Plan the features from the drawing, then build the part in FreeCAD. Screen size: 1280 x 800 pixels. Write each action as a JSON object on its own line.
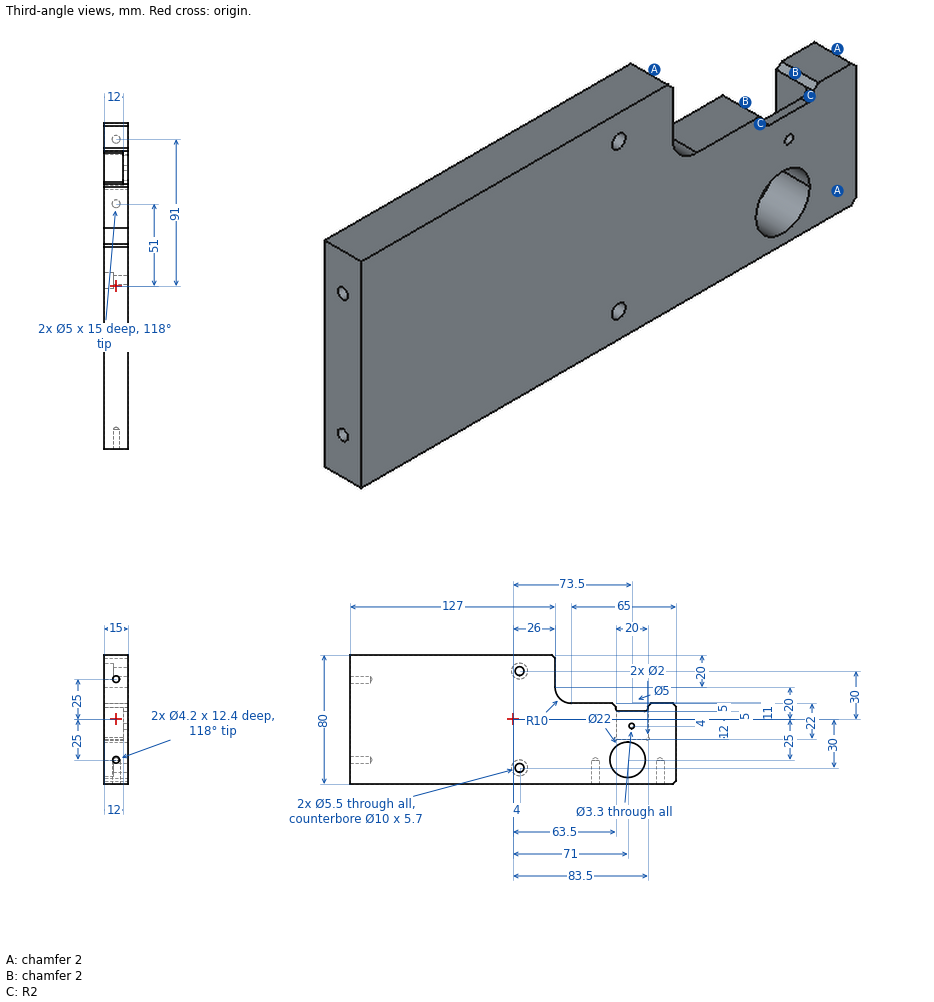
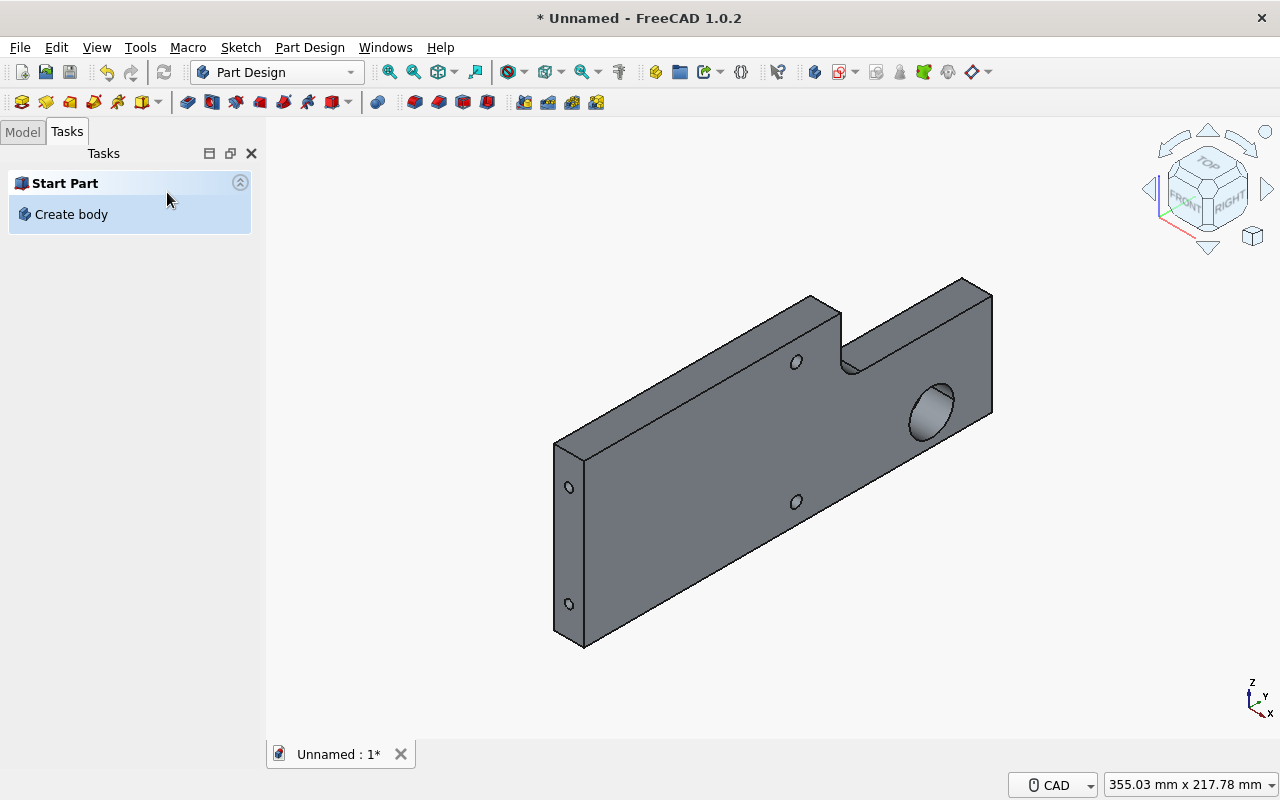
{"action": "key", "text": "2"}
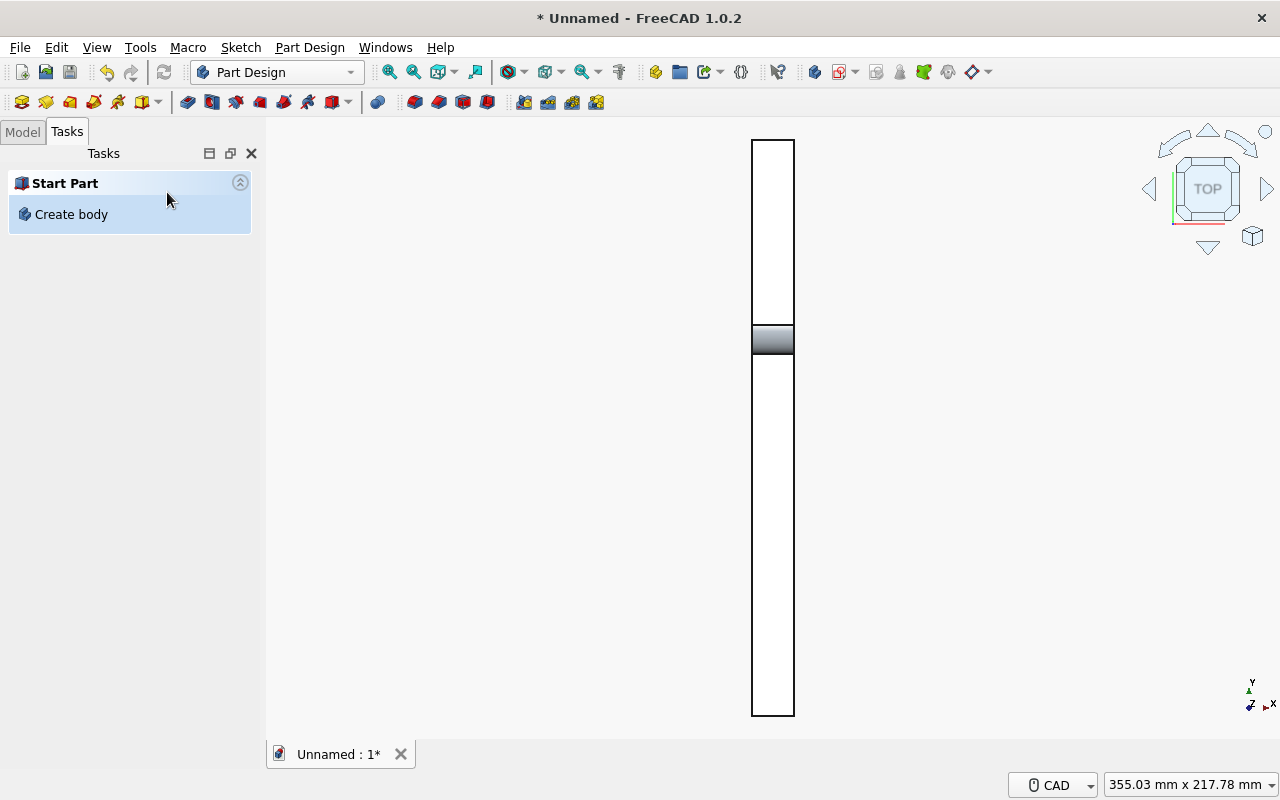
{"action": "left_click", "coordinate": [773, 353]}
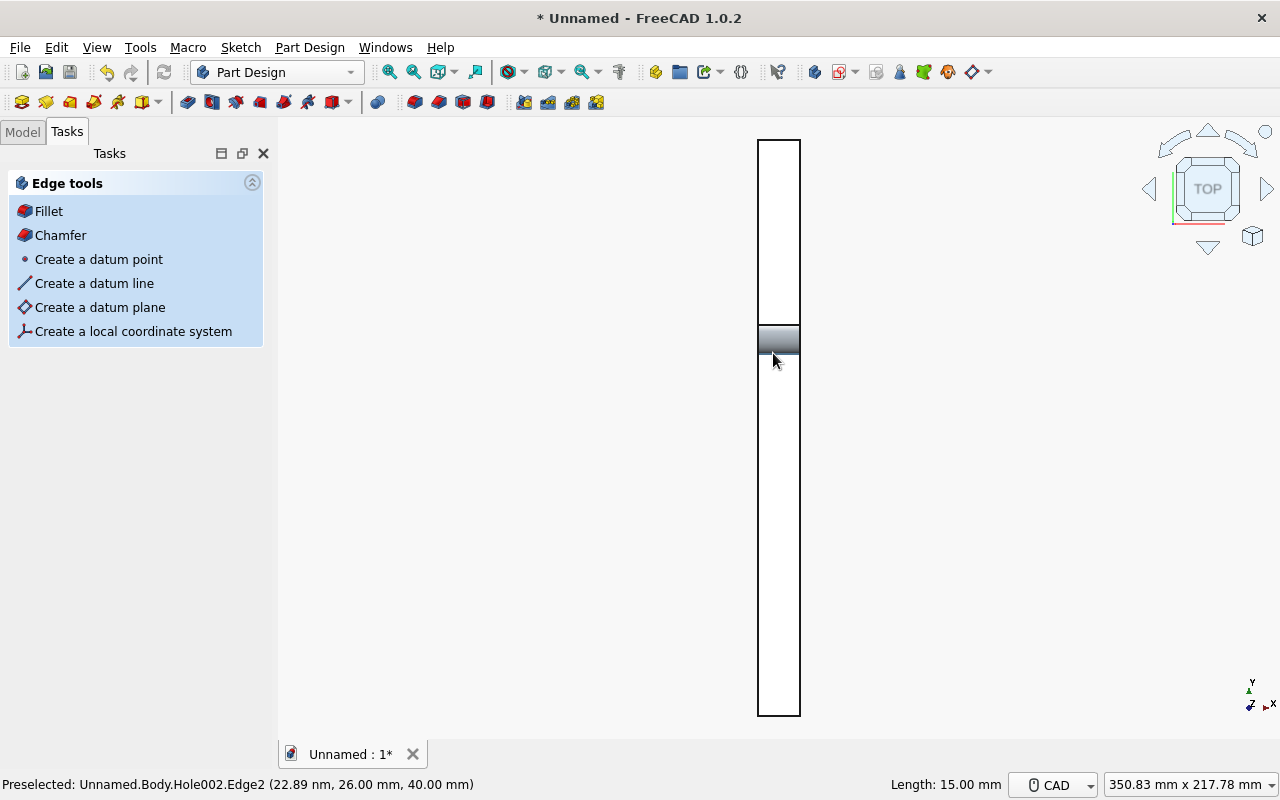
{"action": "key", "text": "1"}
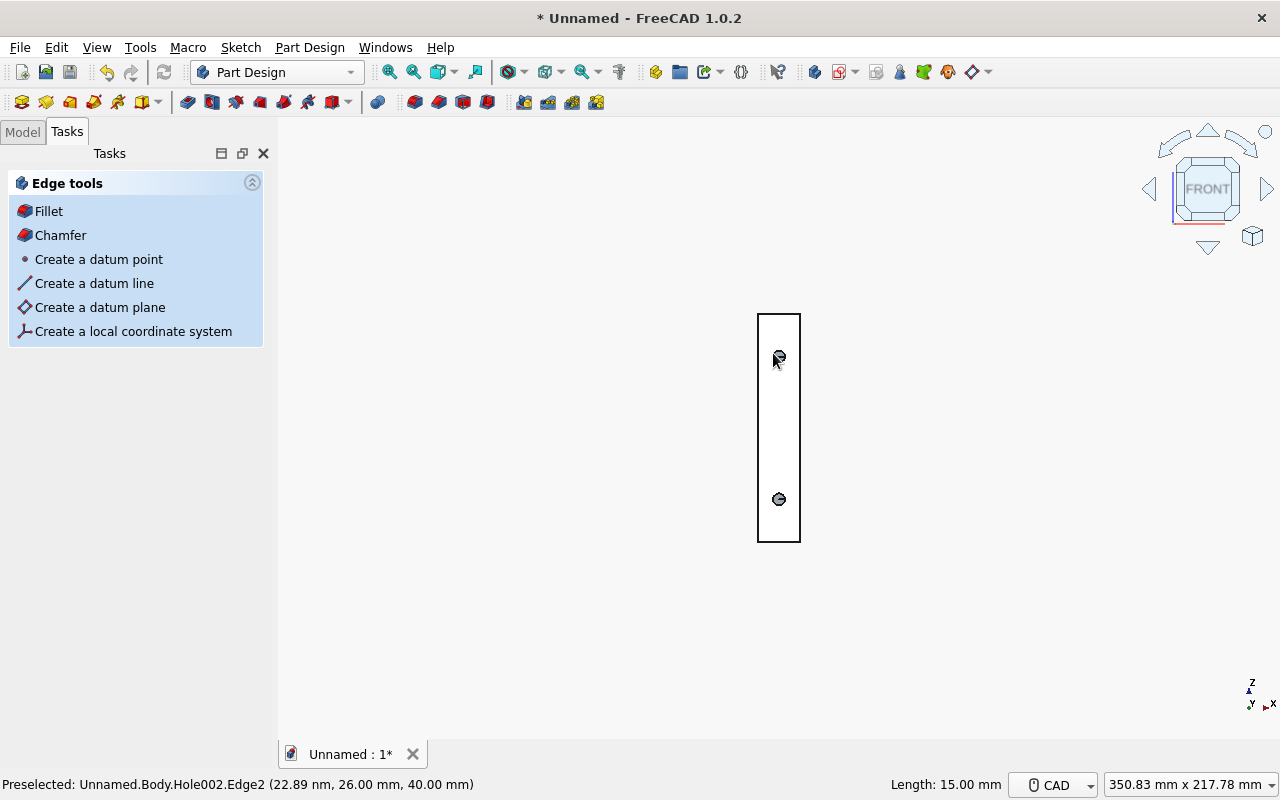
{"action": "left_click", "coordinate": [390, 72]}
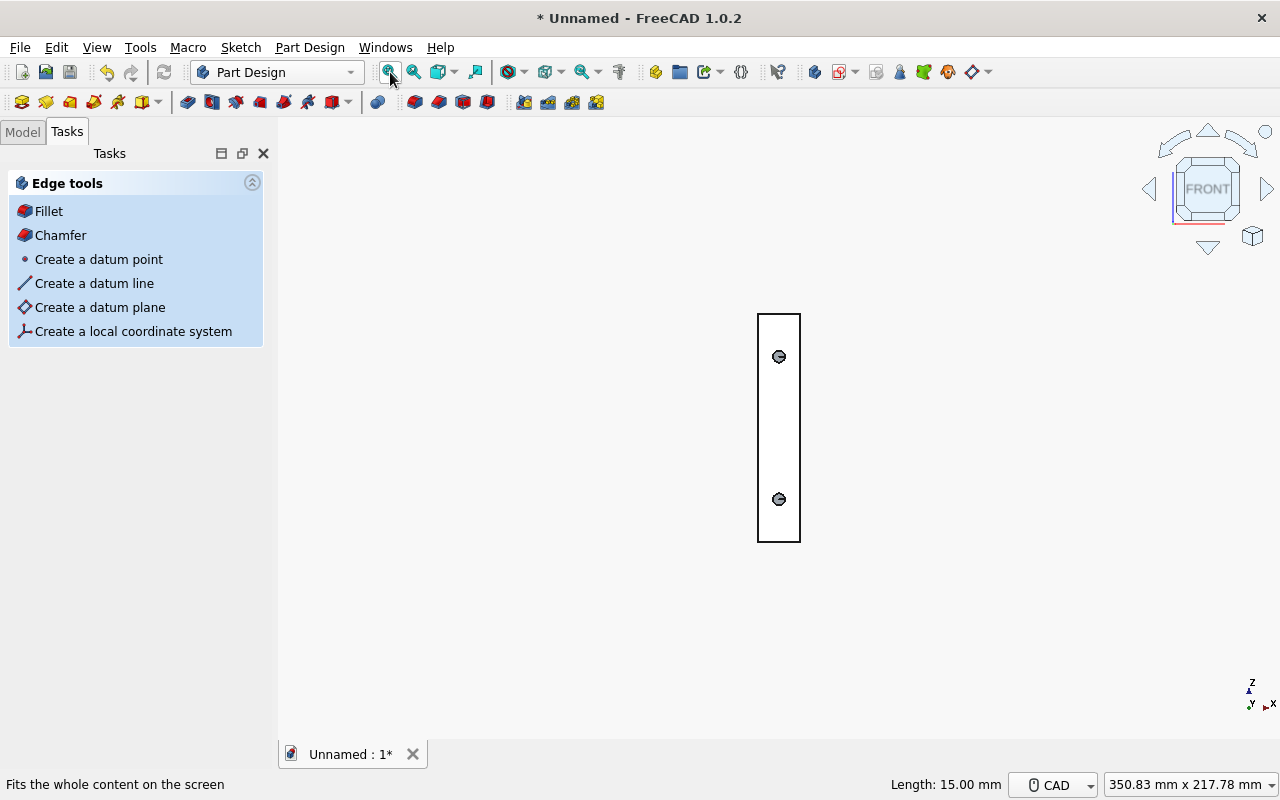
{"action": "key", "text": "3"}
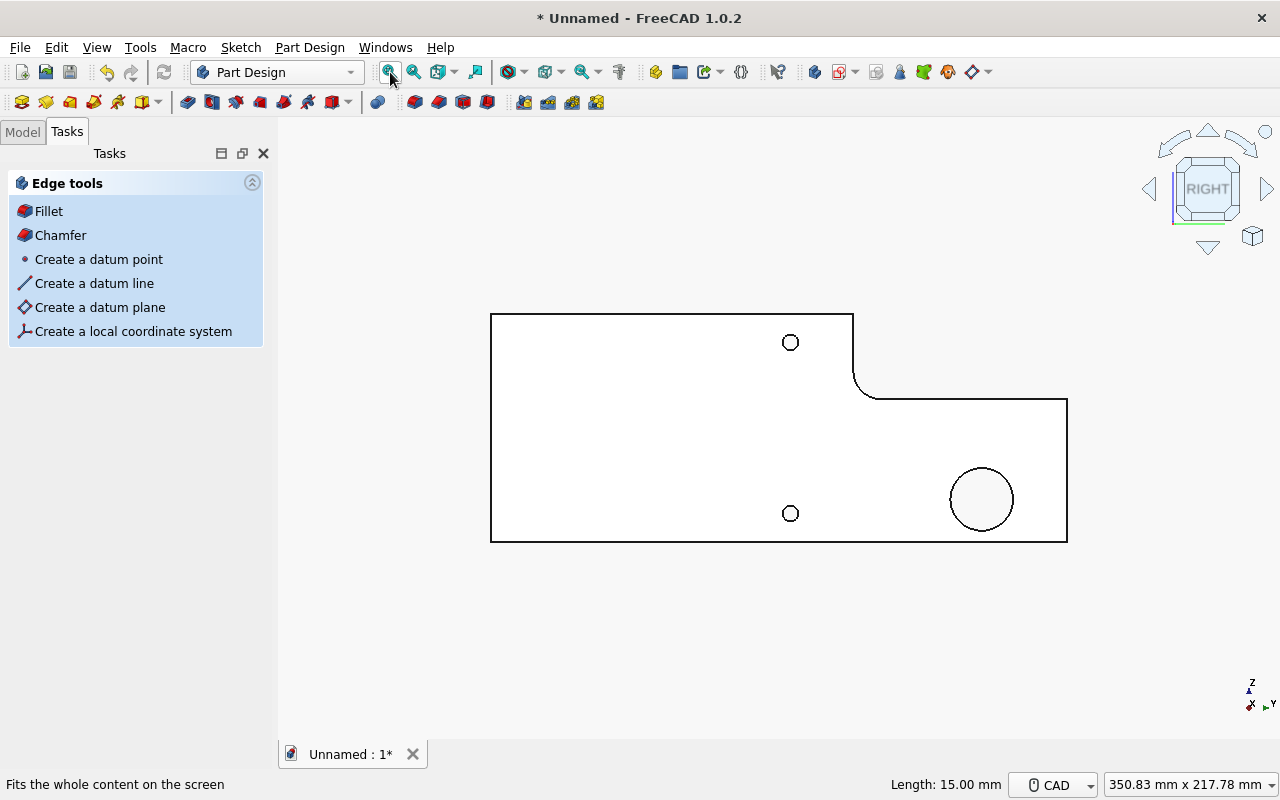
{"action": "key", "text": "5"}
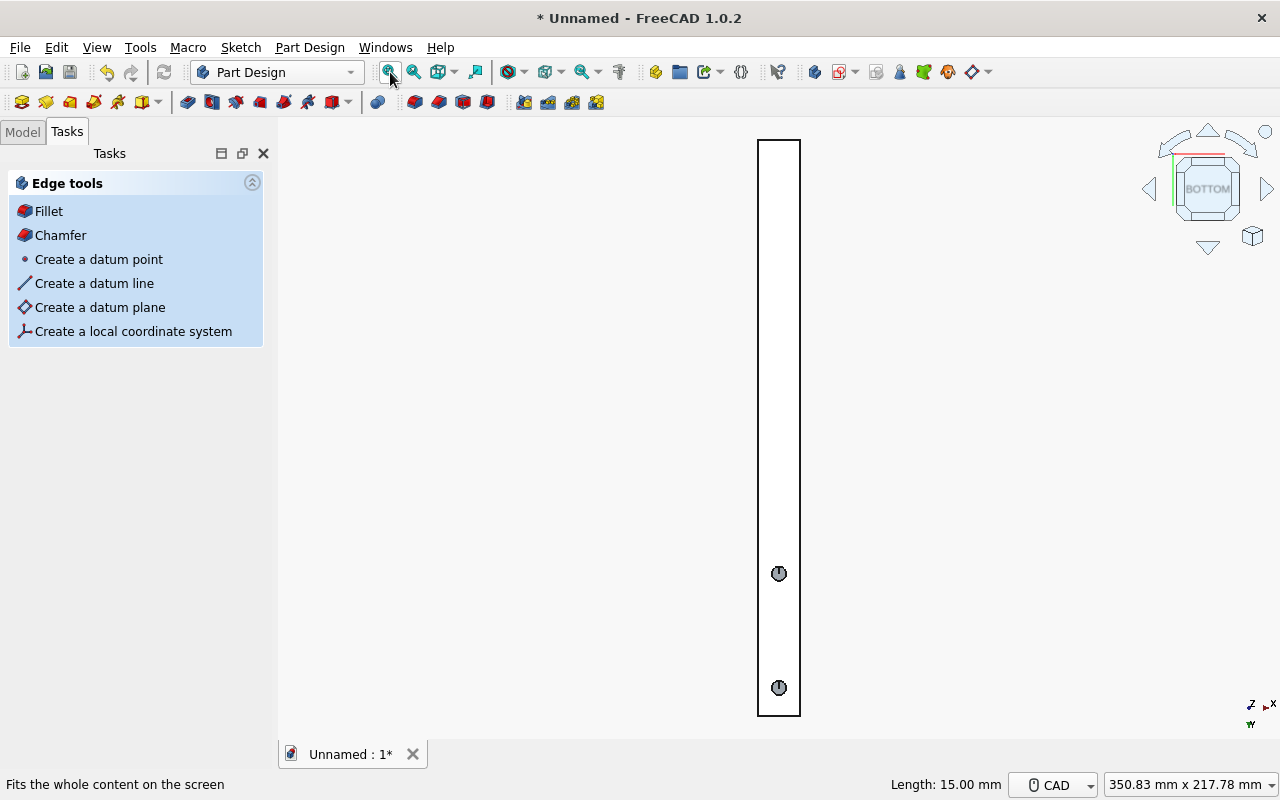
{"action": "key", "text": "4"}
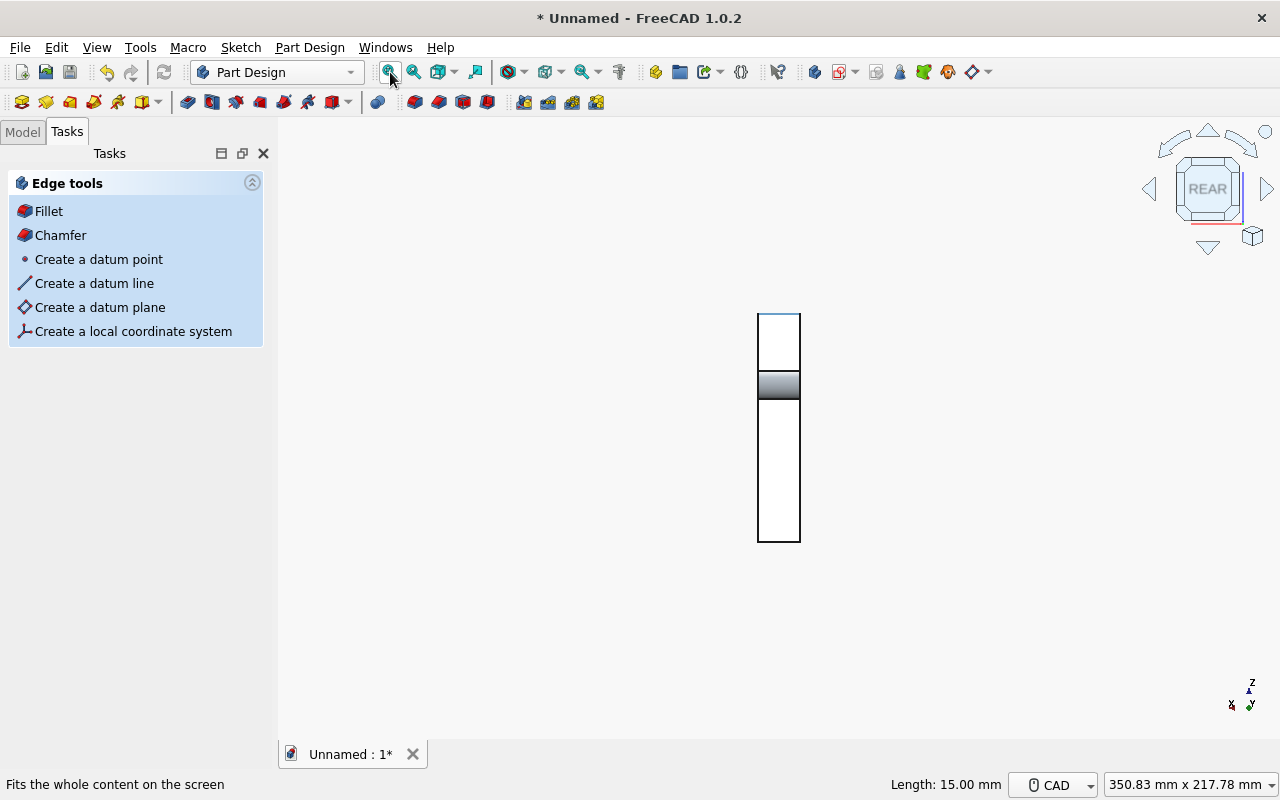
{"action": "left_click", "coordinate": [390, 72]}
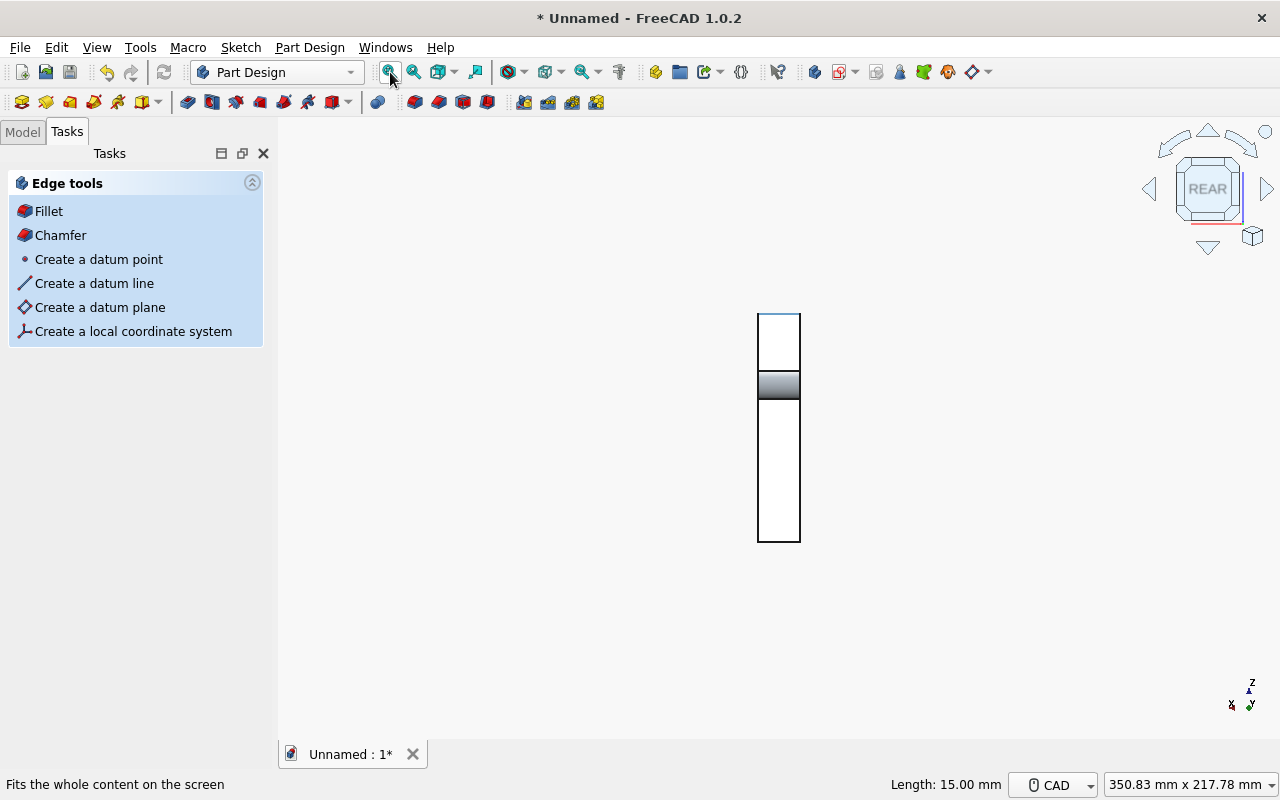
{"action": "left_click", "coordinate": [779, 398], "text": "ctrl"}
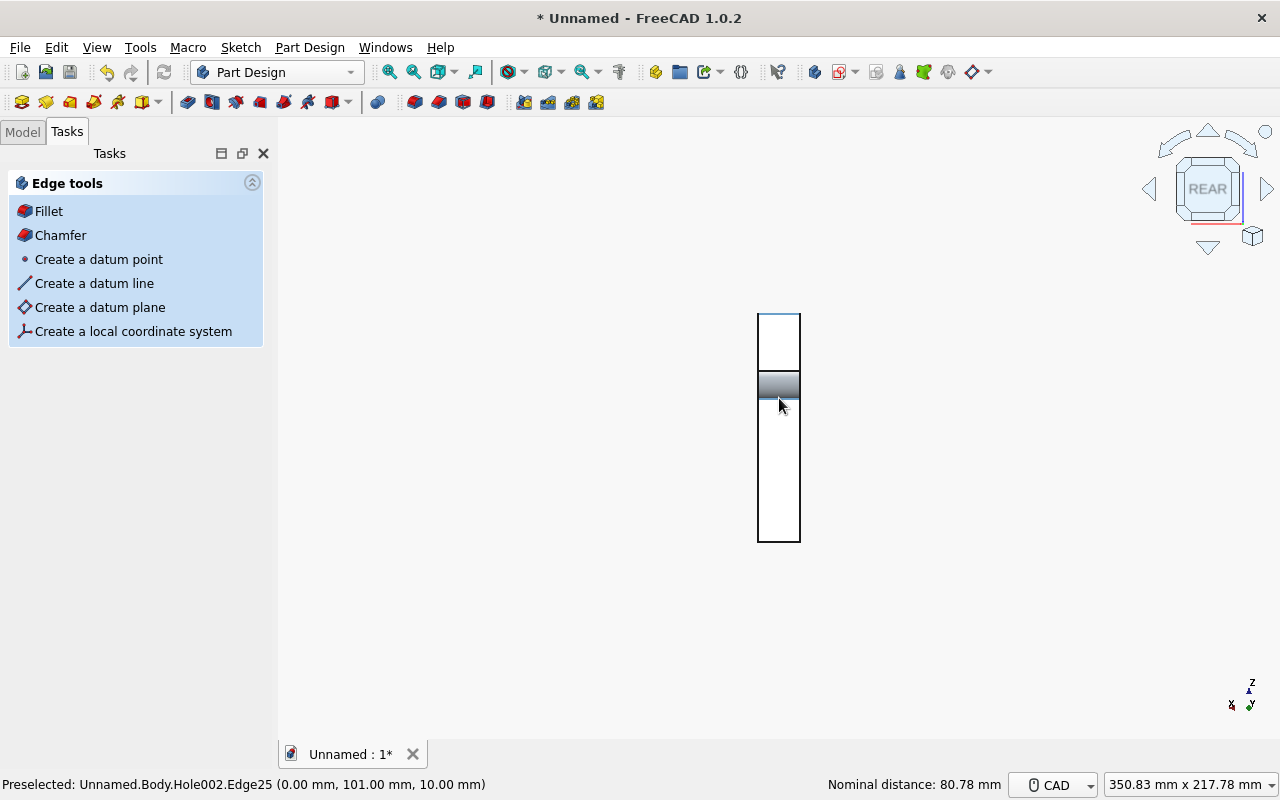
{"action": "left_click", "coordinate": [779, 541], "text": "ctrl"}